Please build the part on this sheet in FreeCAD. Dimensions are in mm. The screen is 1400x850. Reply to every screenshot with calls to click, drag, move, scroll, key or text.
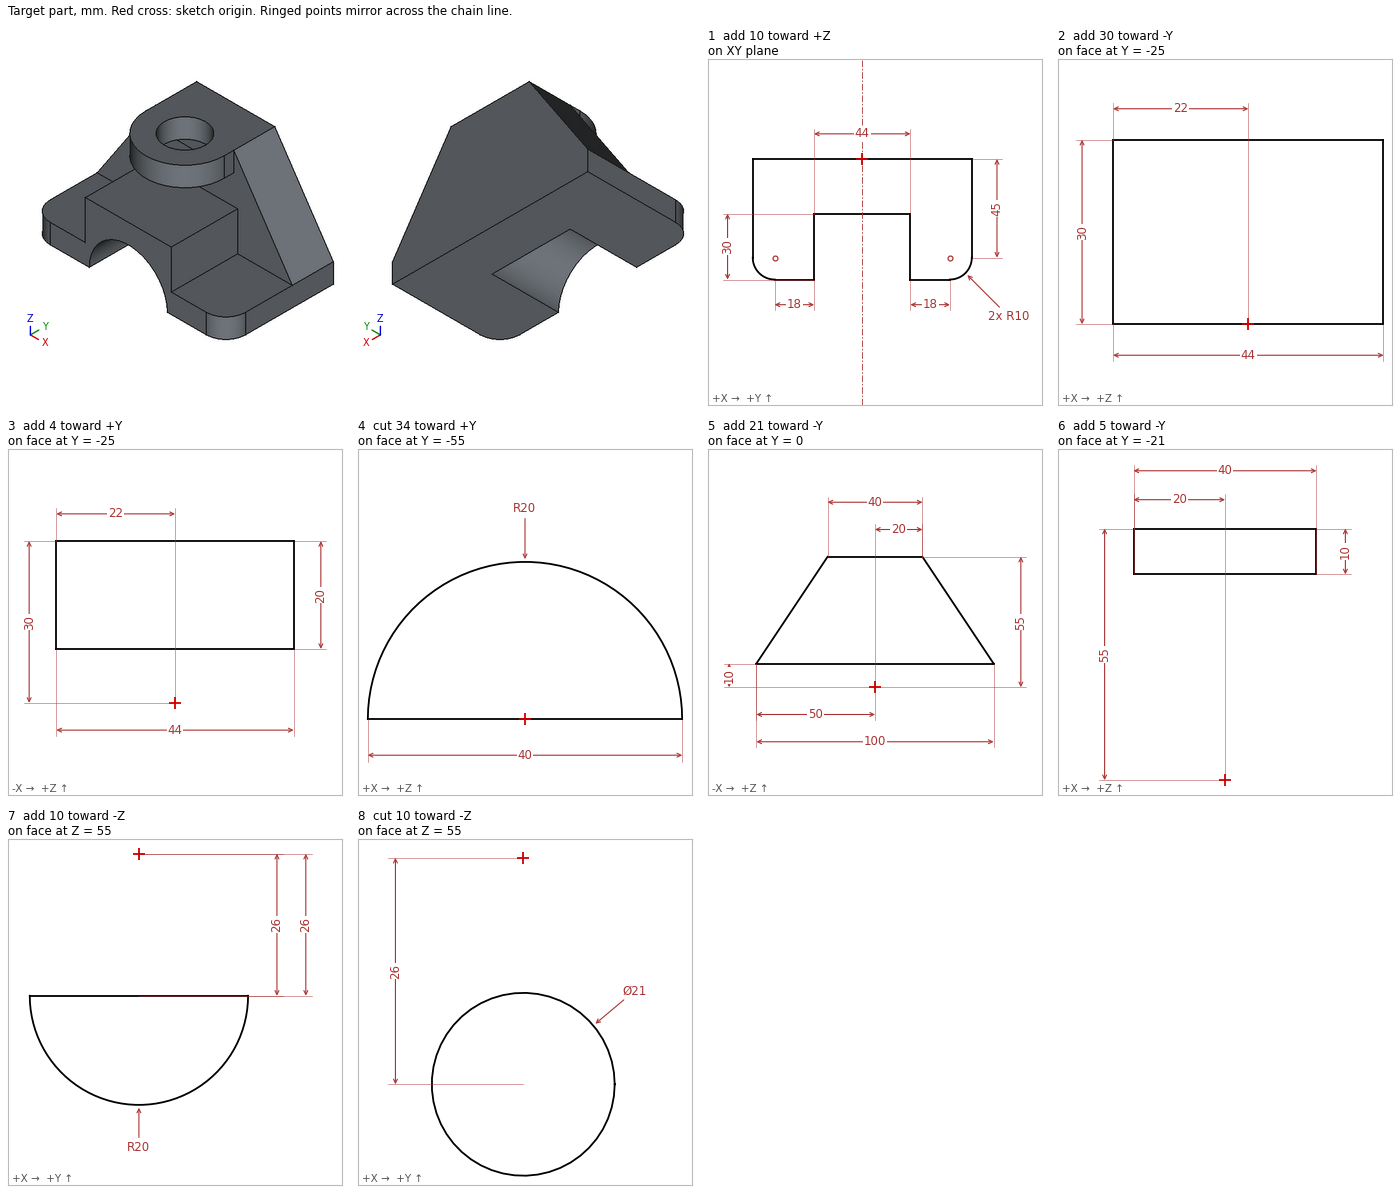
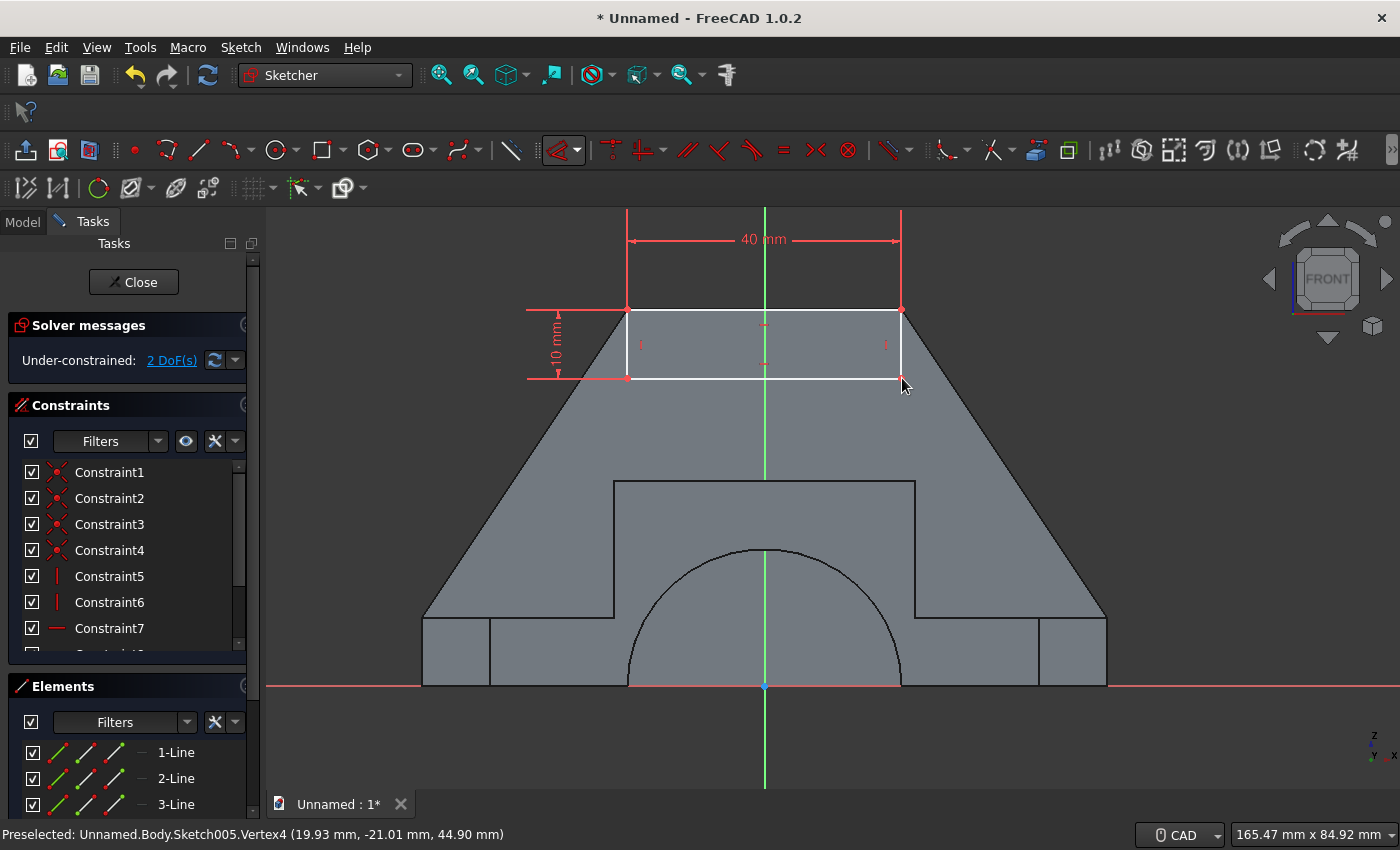
click(627, 310)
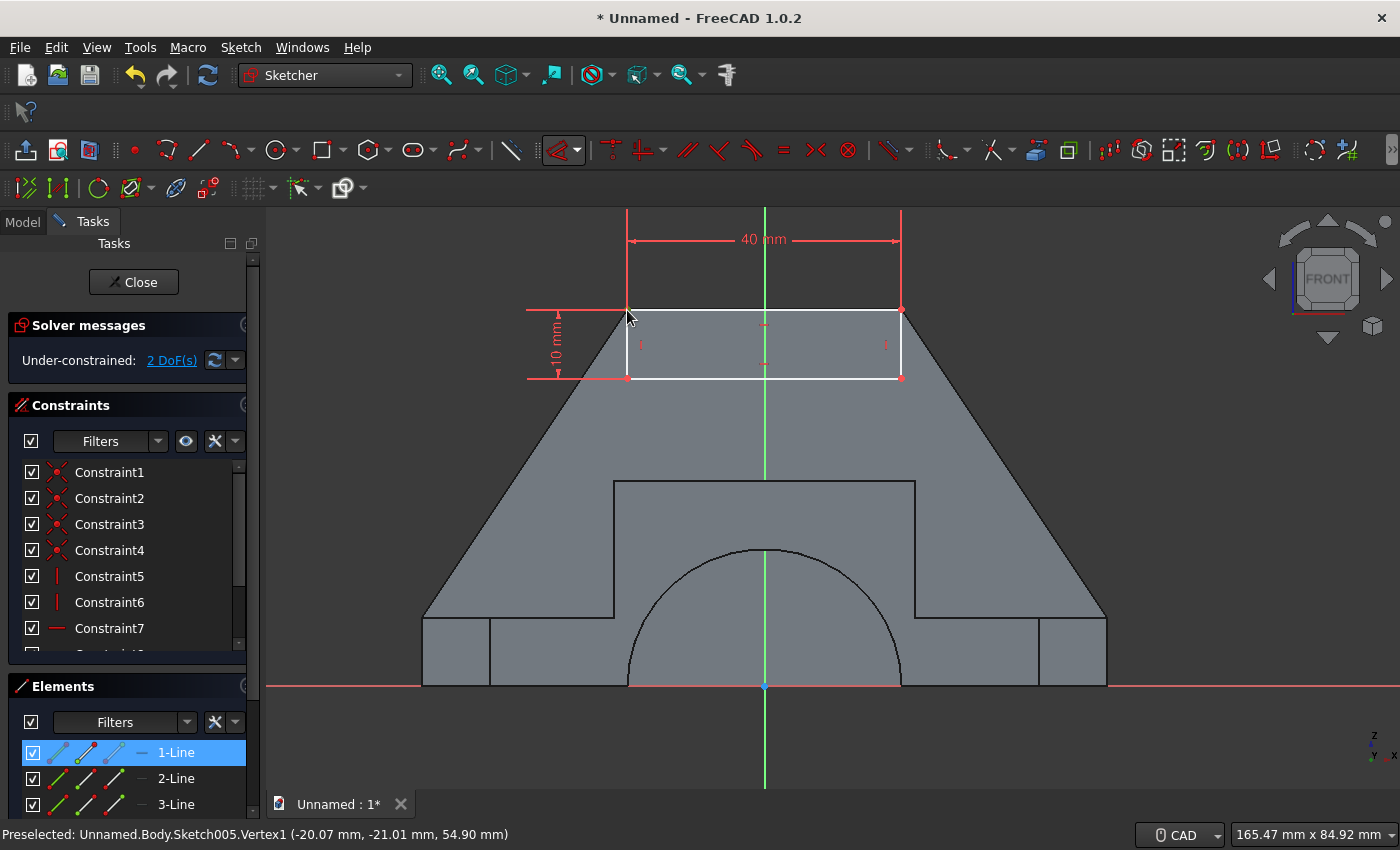
click(580, 150)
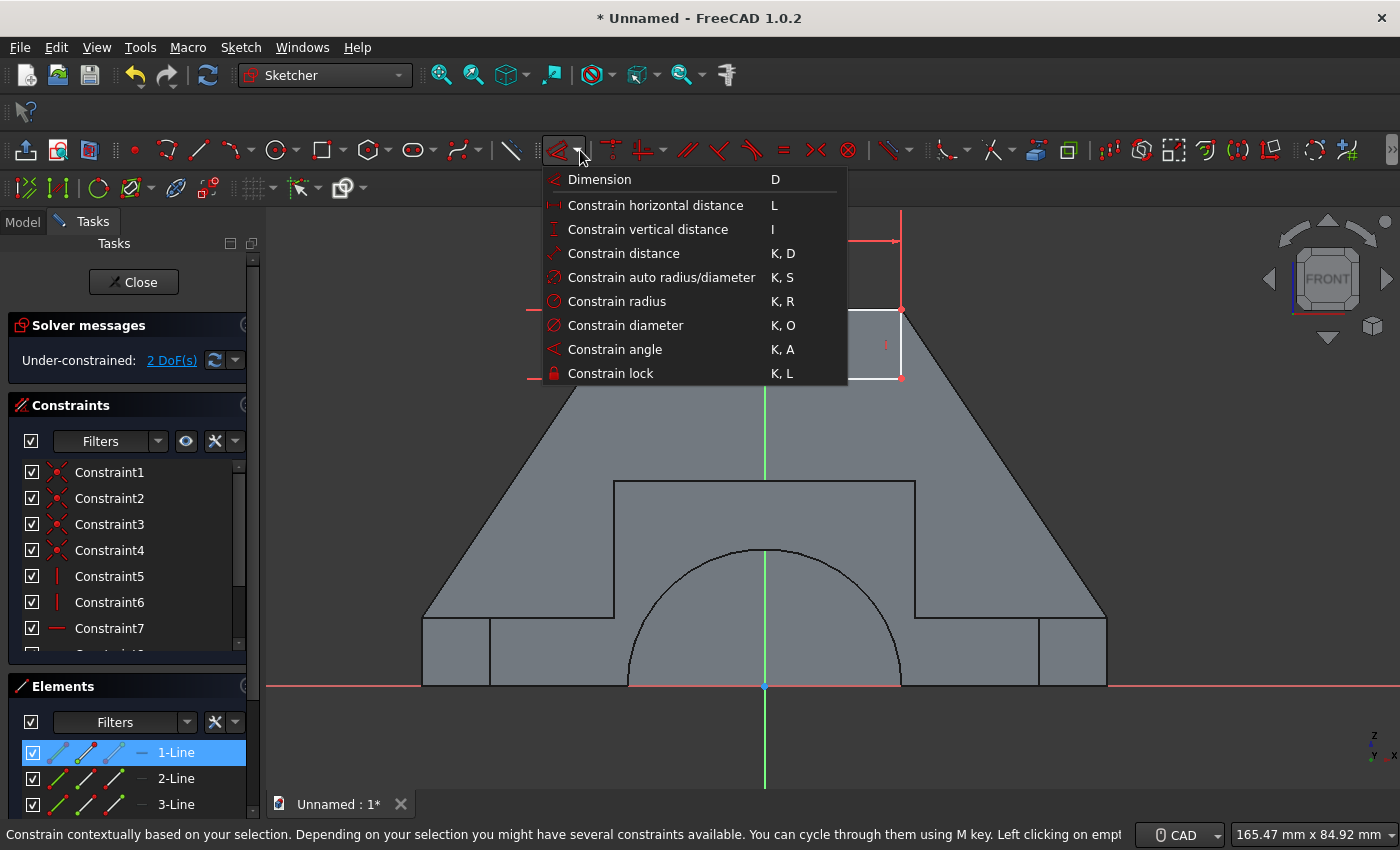
click(695, 205)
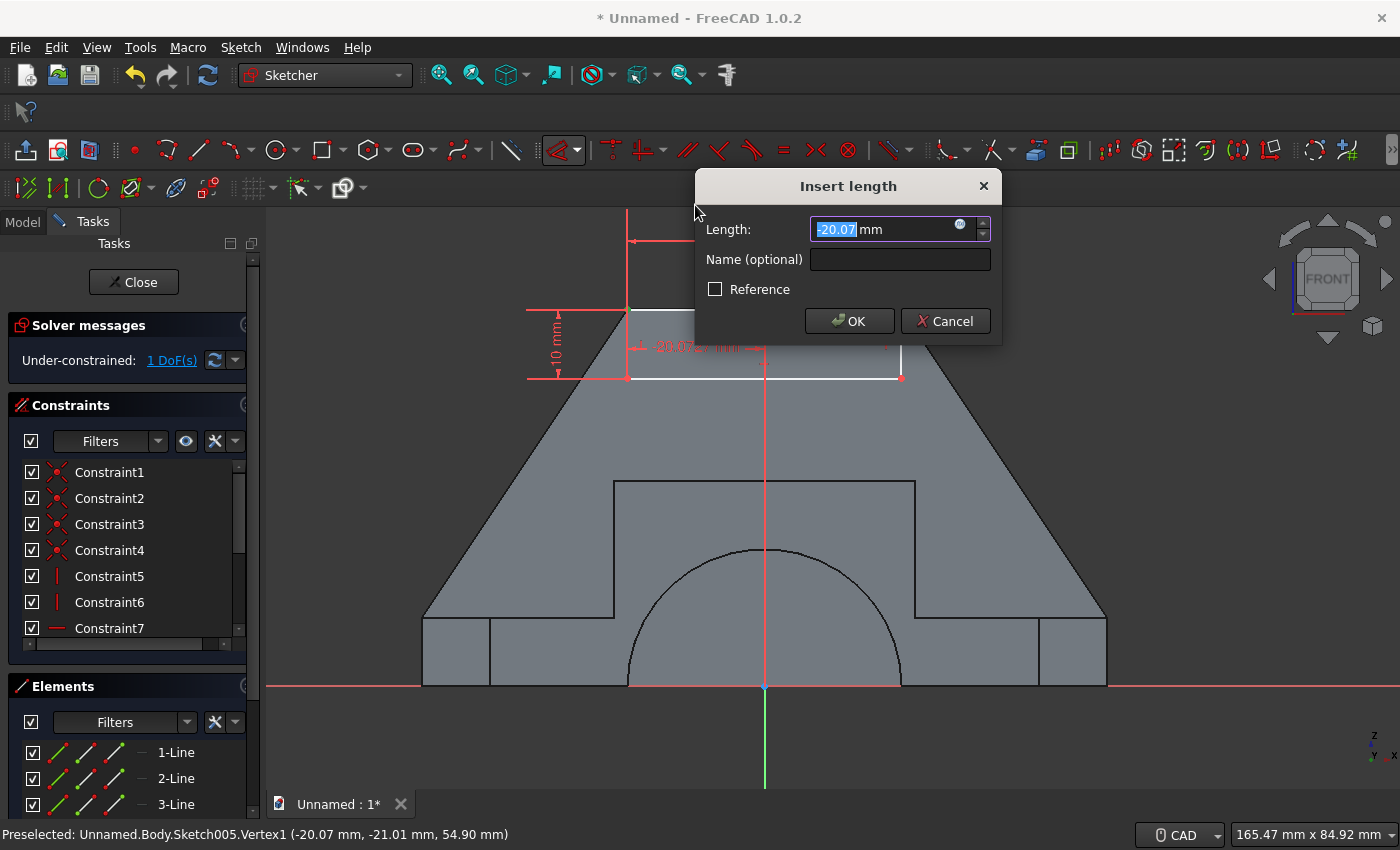
text(-20)
key(Return)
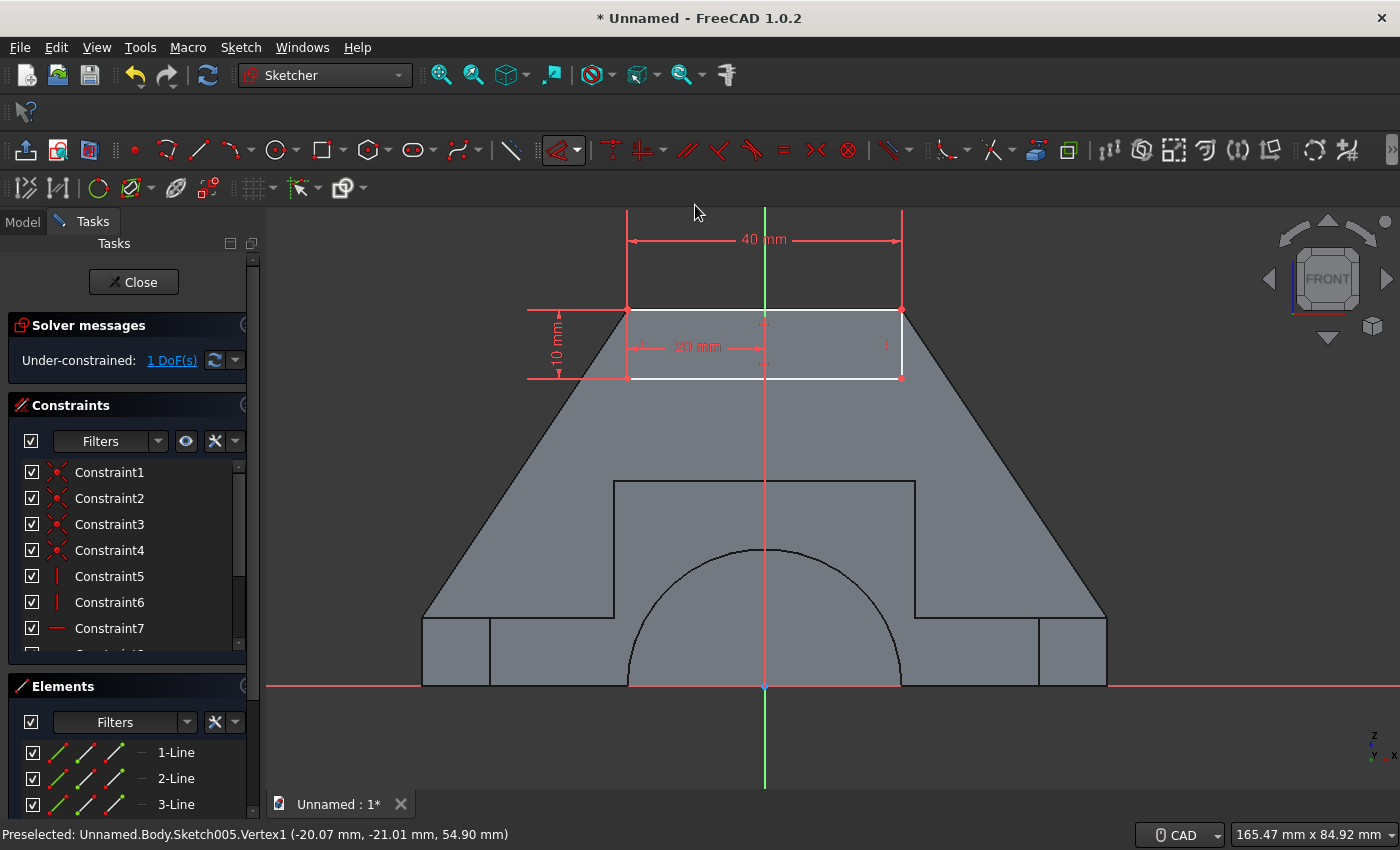
click(627, 310)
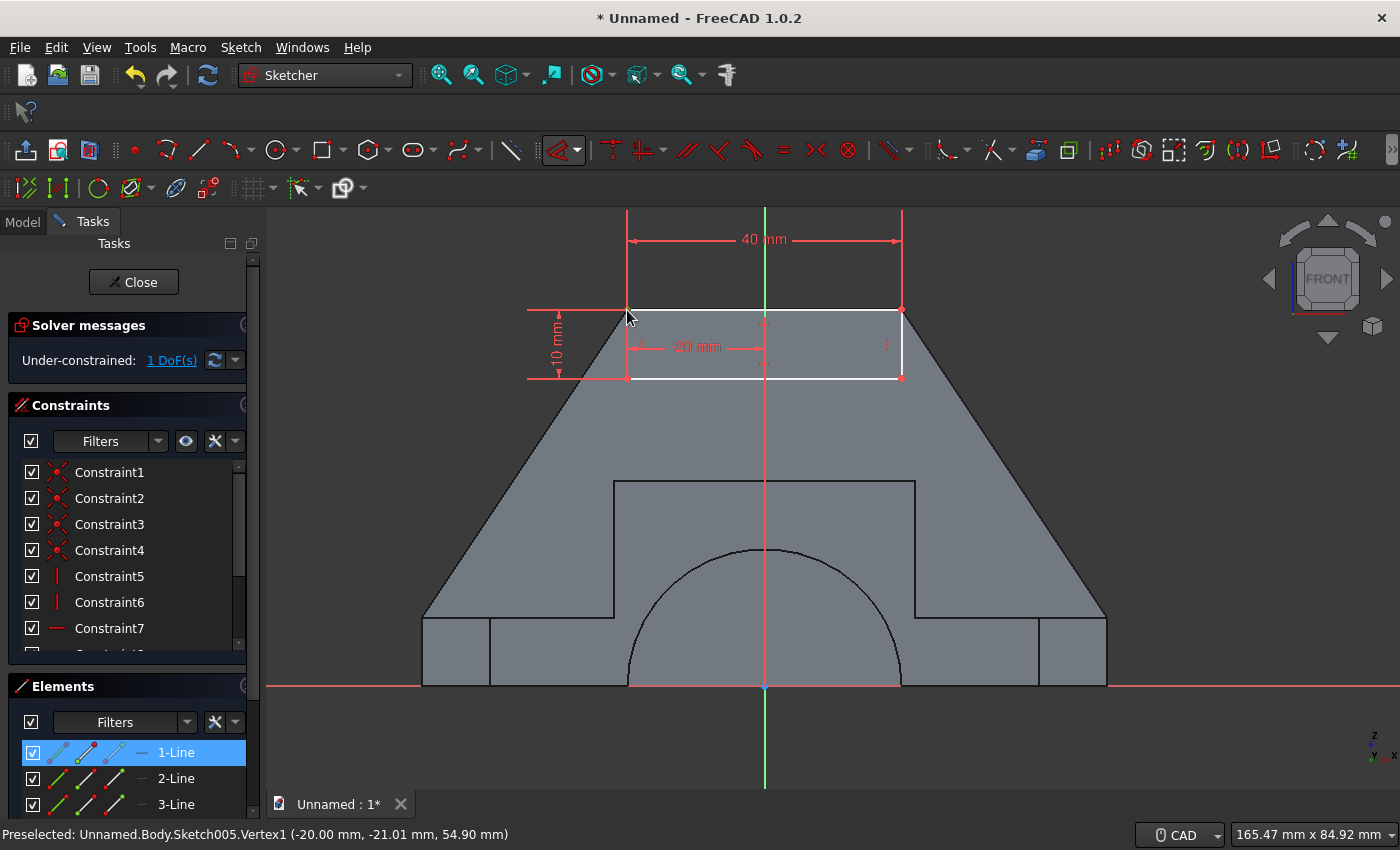
key(i)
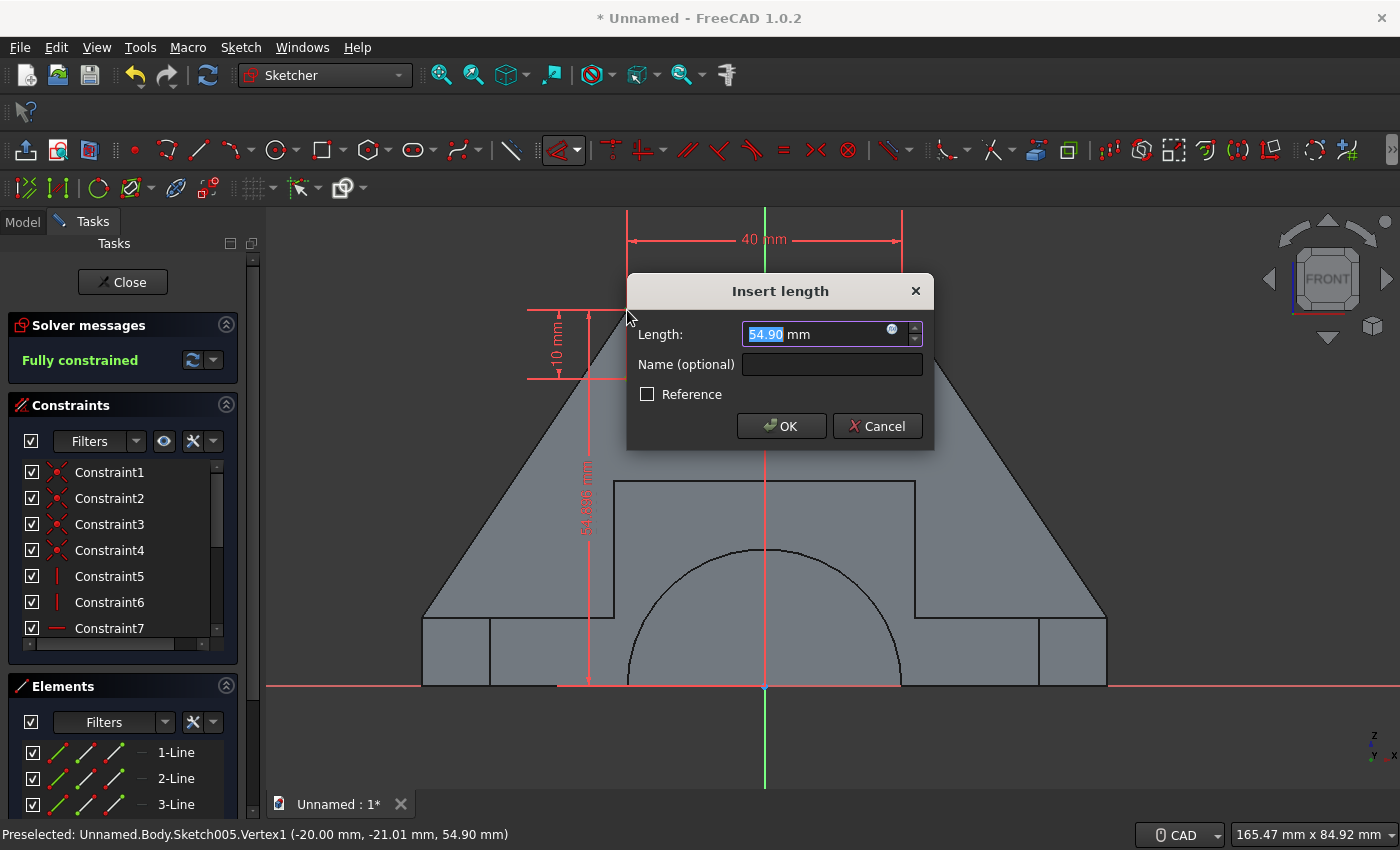
text(55)
key(Return)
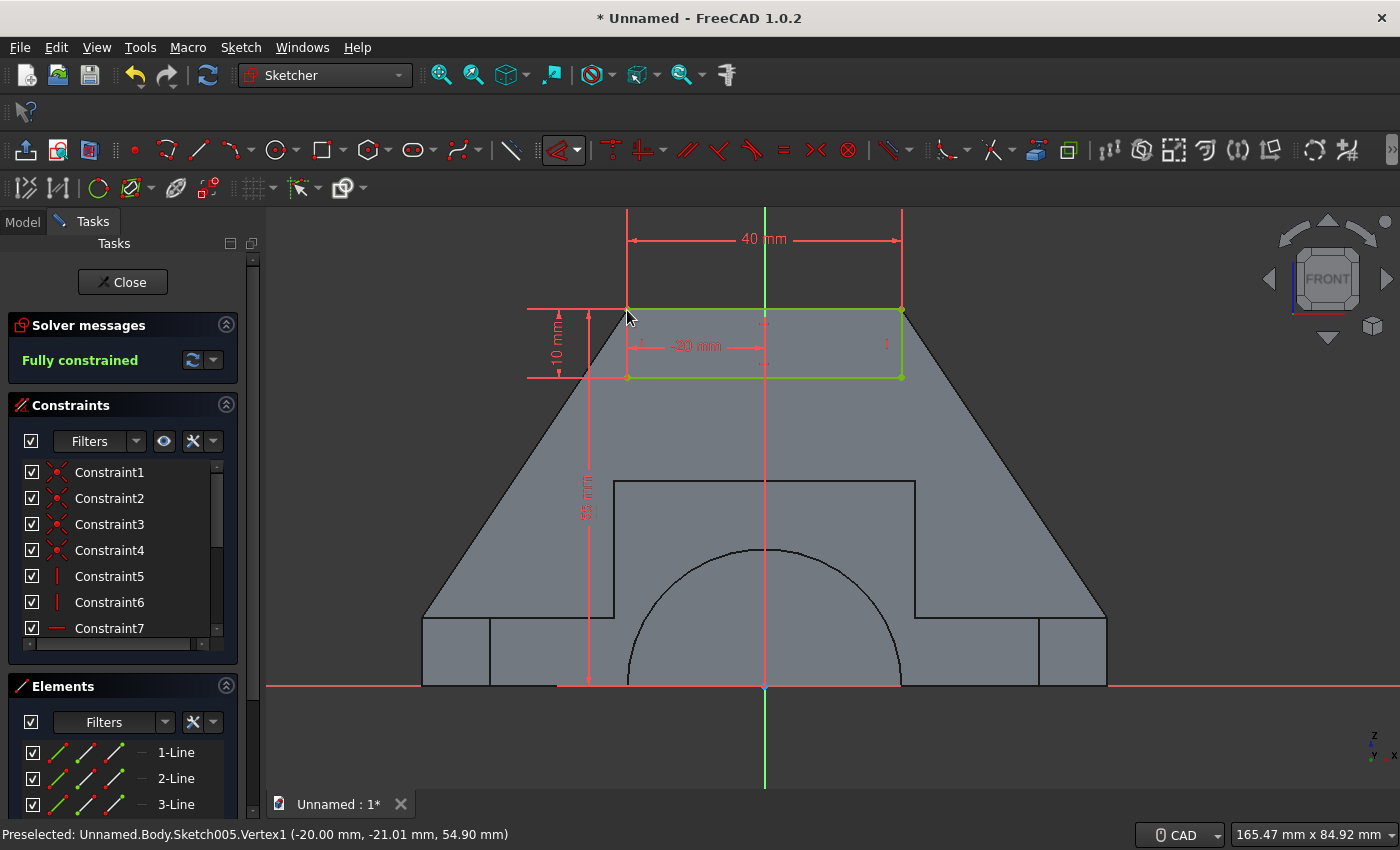
click(123, 282)